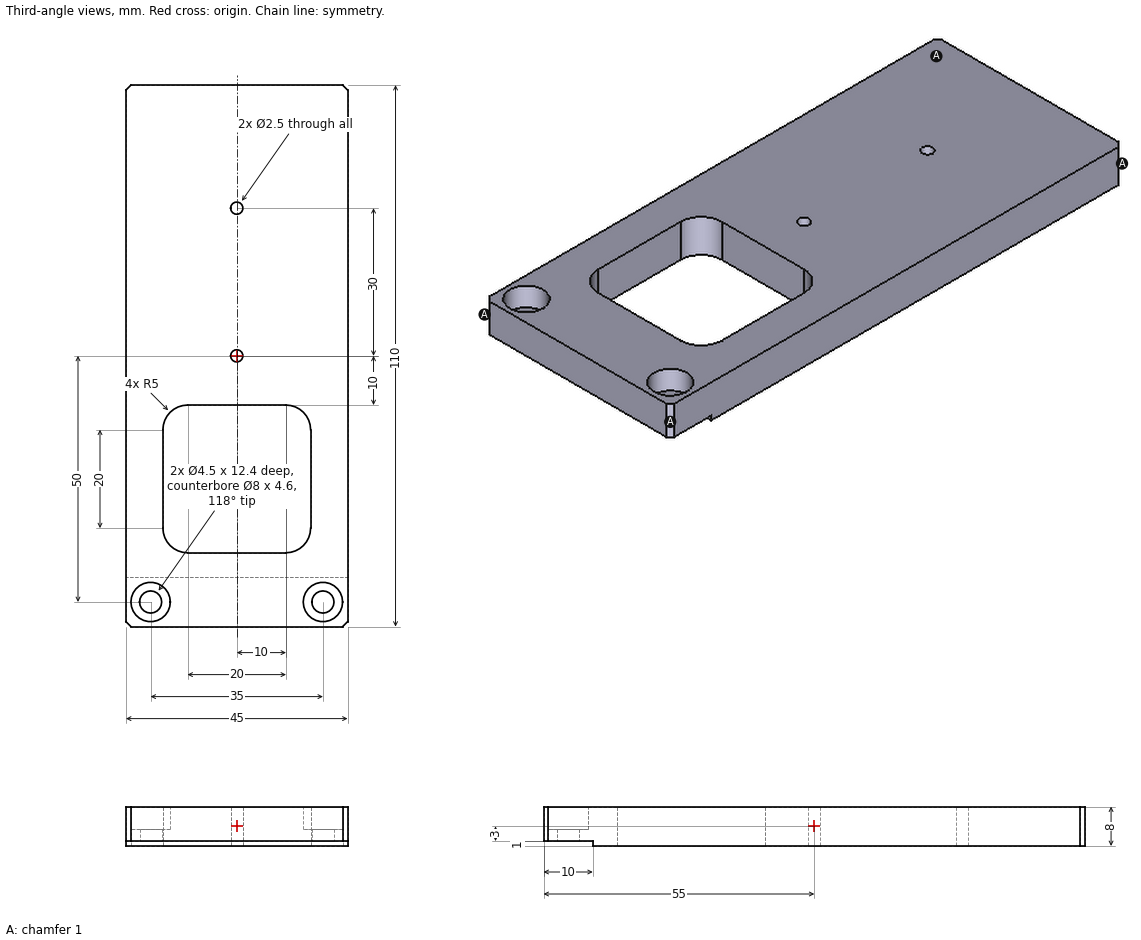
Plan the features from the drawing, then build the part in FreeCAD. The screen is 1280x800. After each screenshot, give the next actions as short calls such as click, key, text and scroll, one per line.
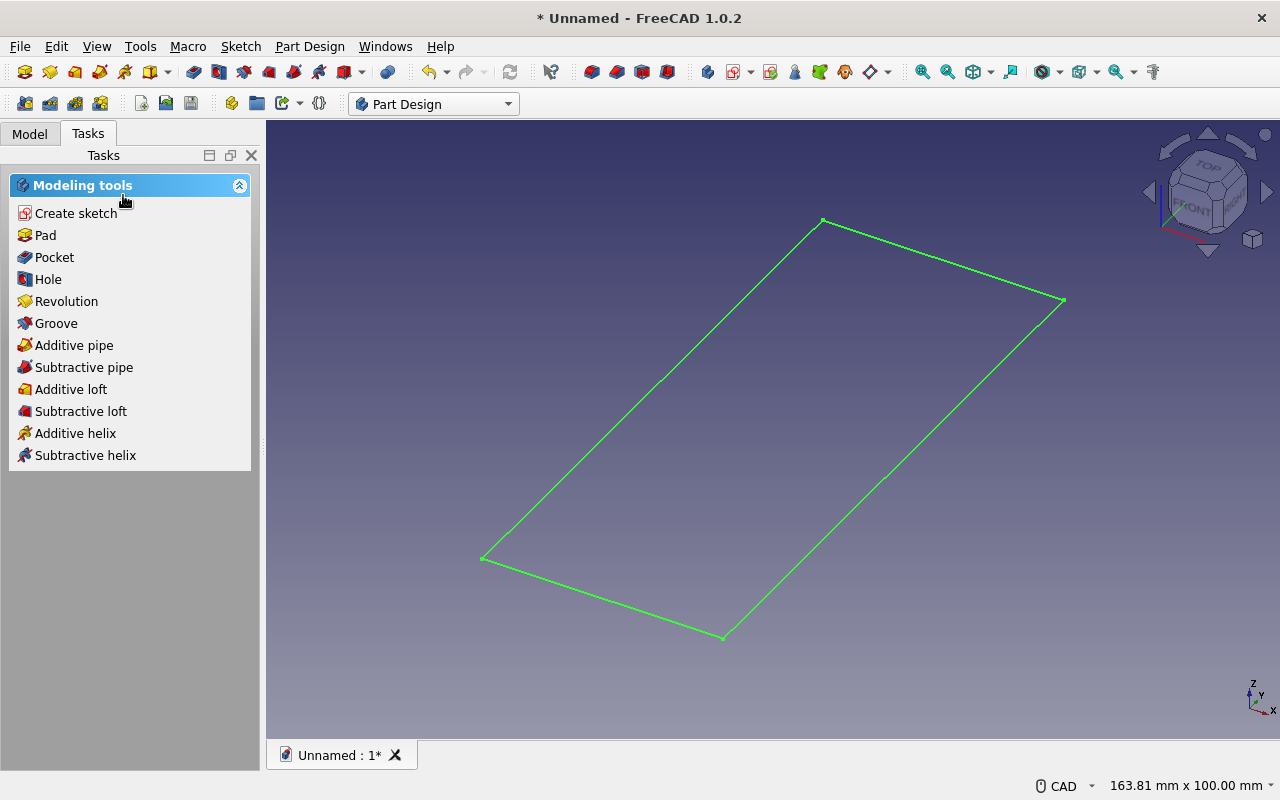
click(25, 72)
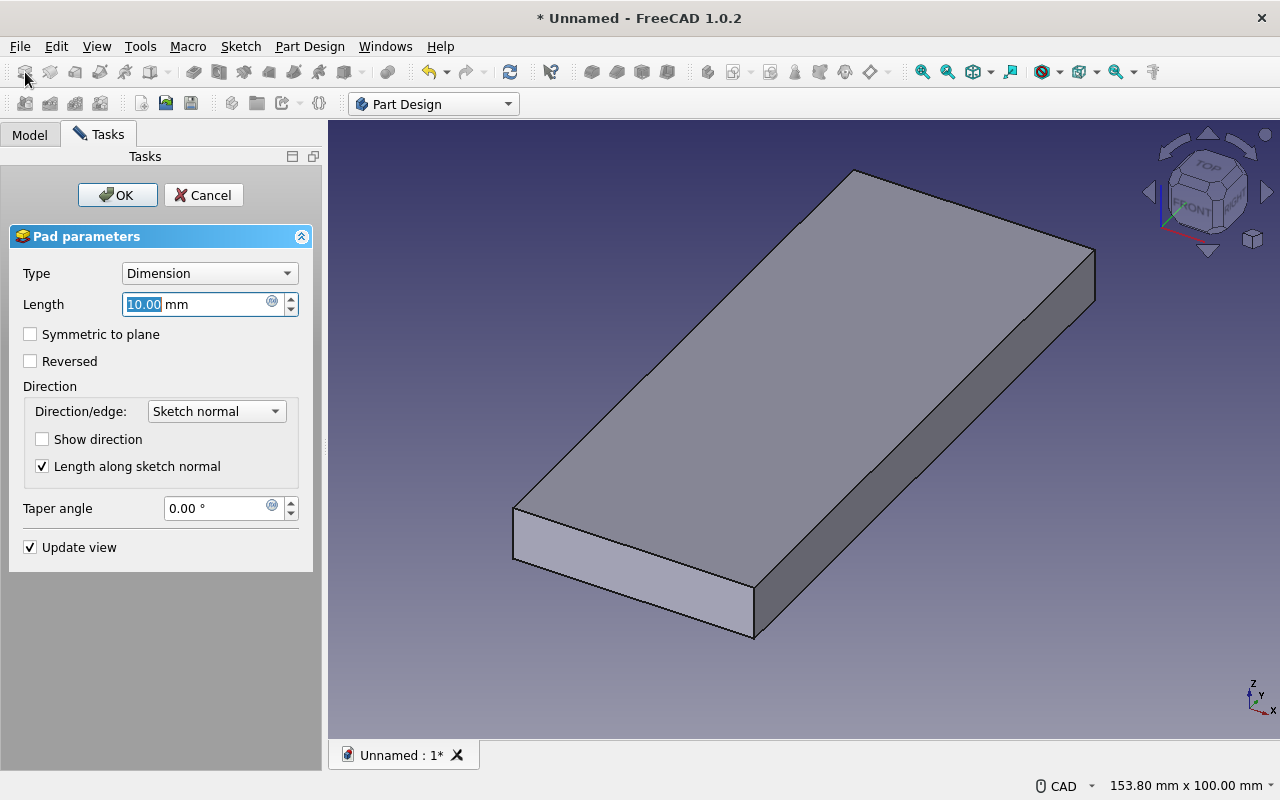
text(8)
key(Tab)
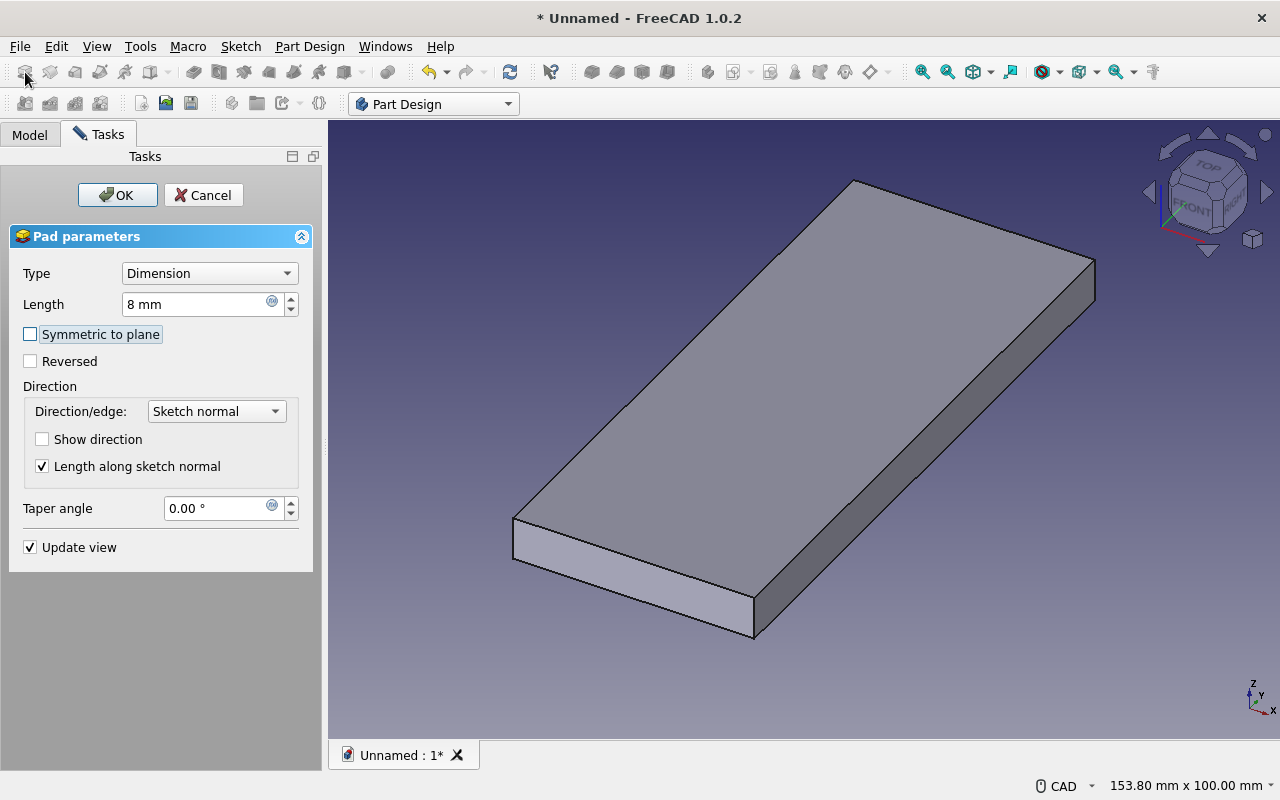
click(31, 334)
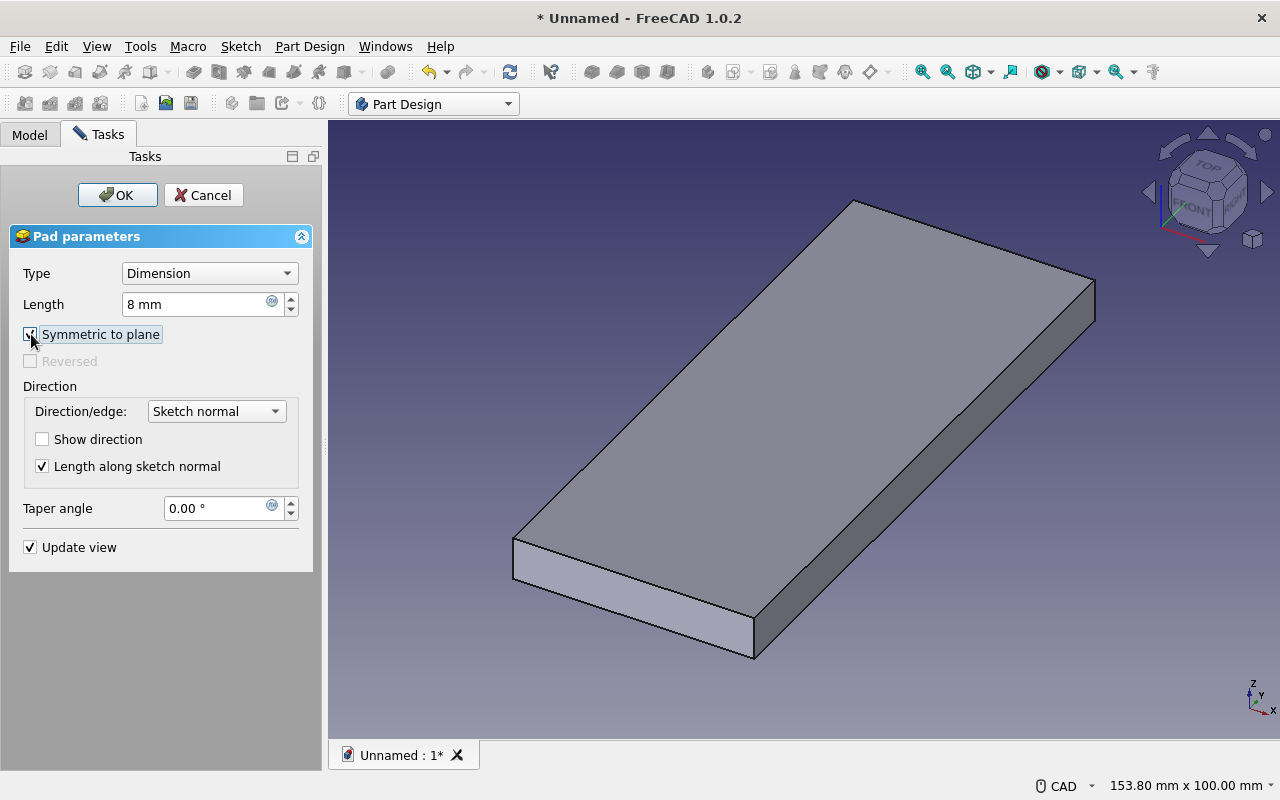
click(118, 195)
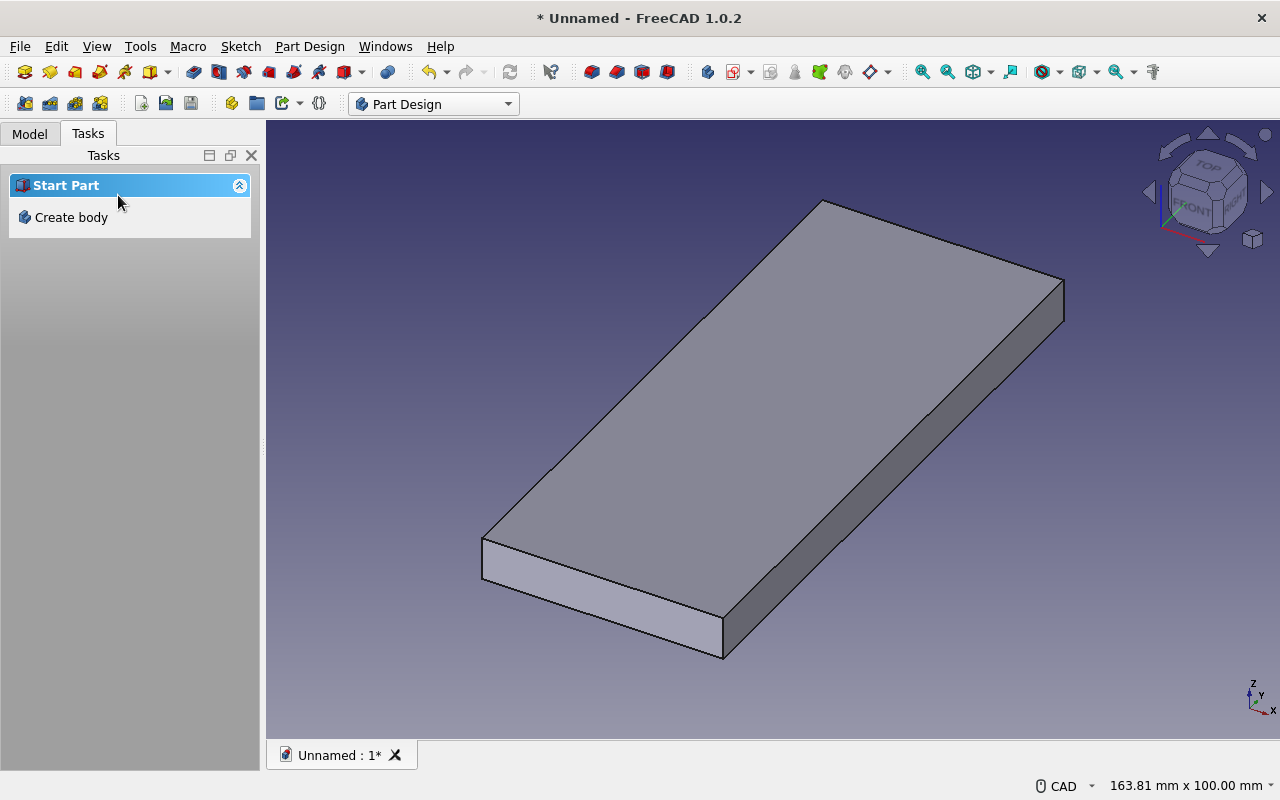
click(870, 312)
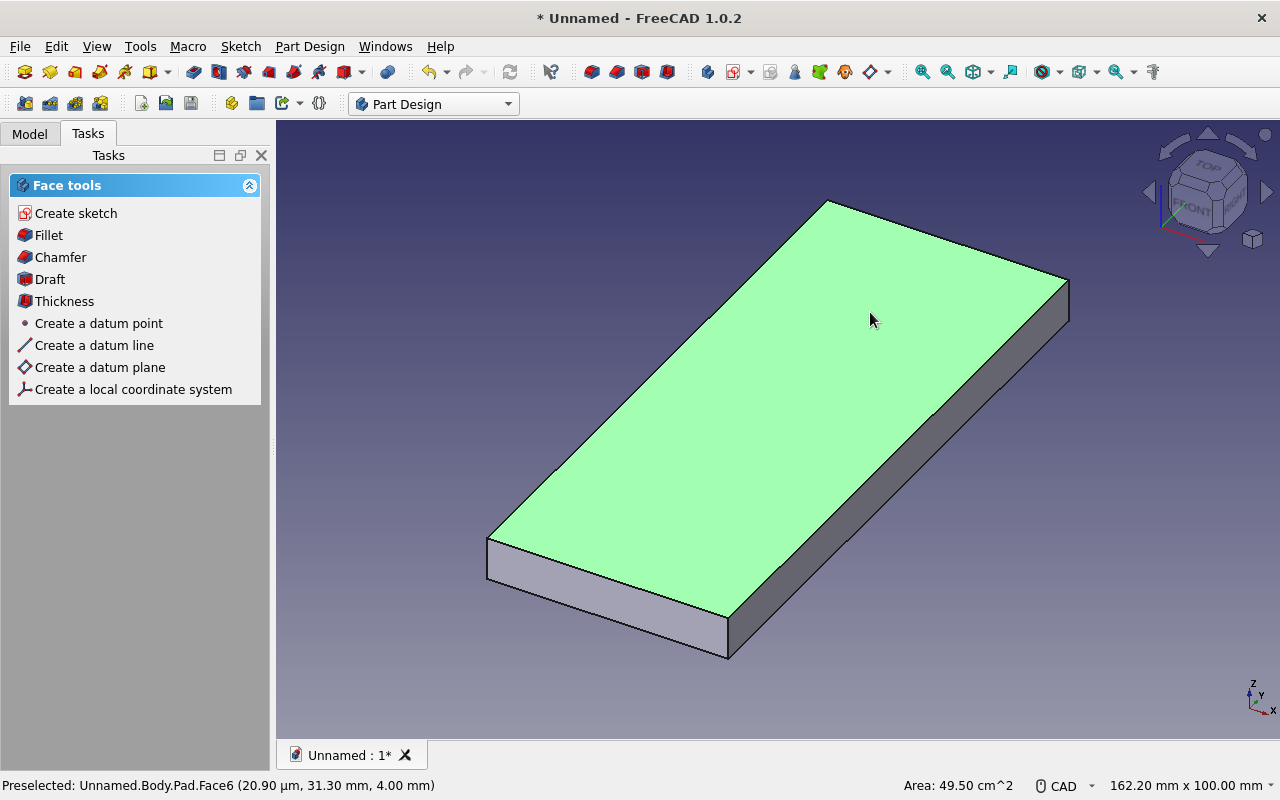
click(732, 72)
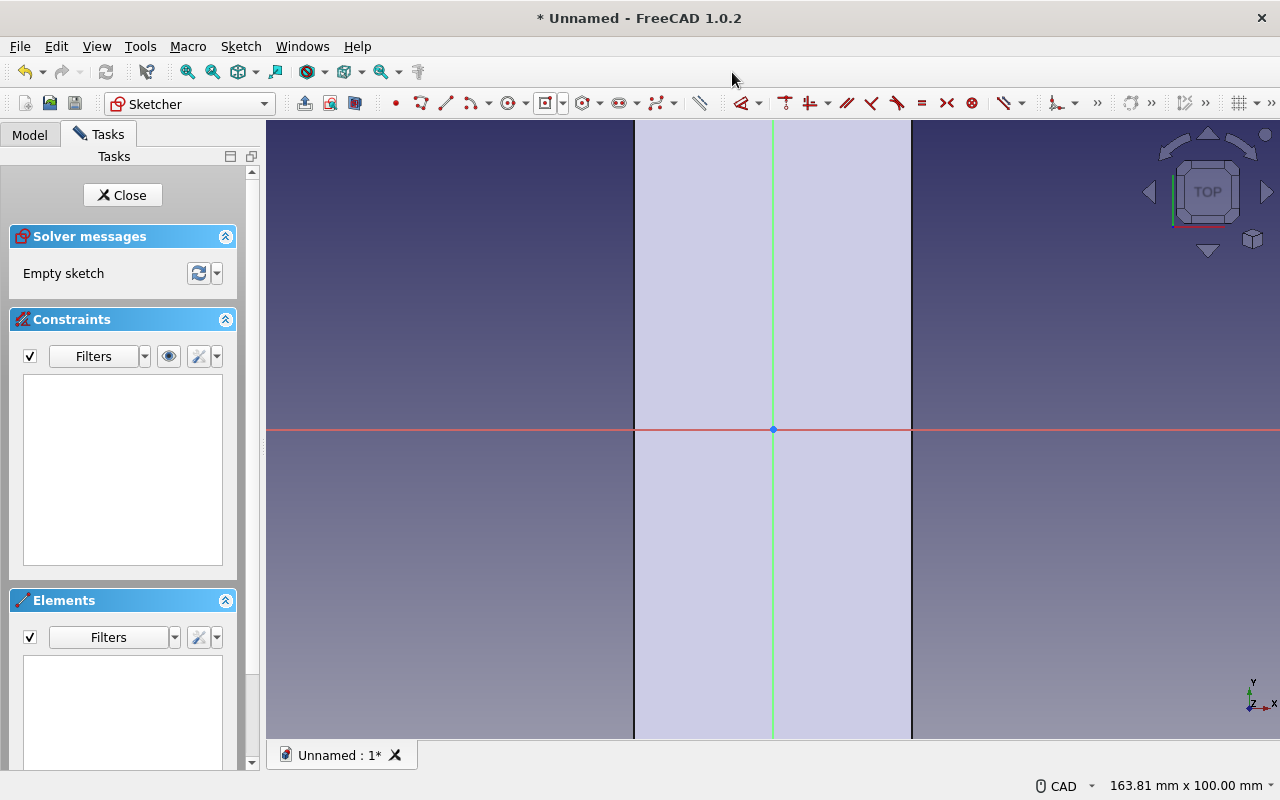
scroll(395, 148, down, 1)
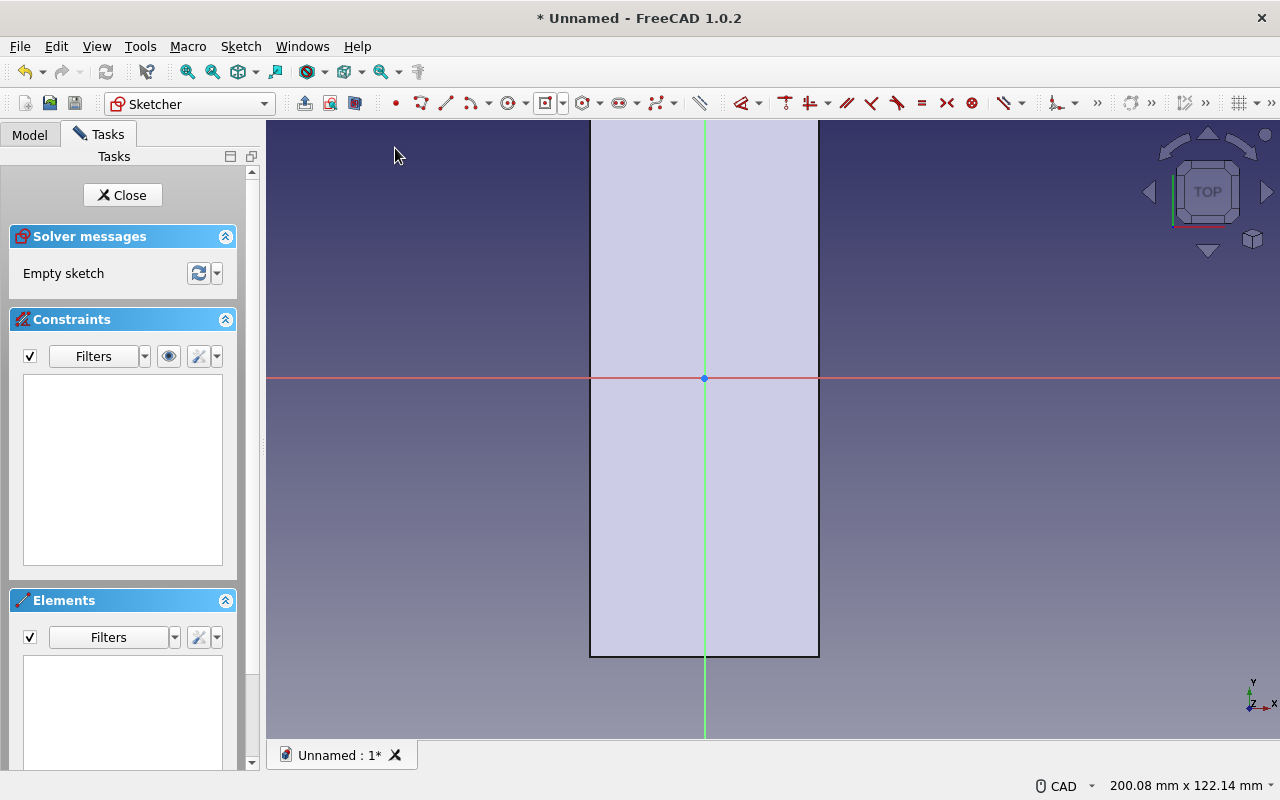
scroll(705, 676, up, 2)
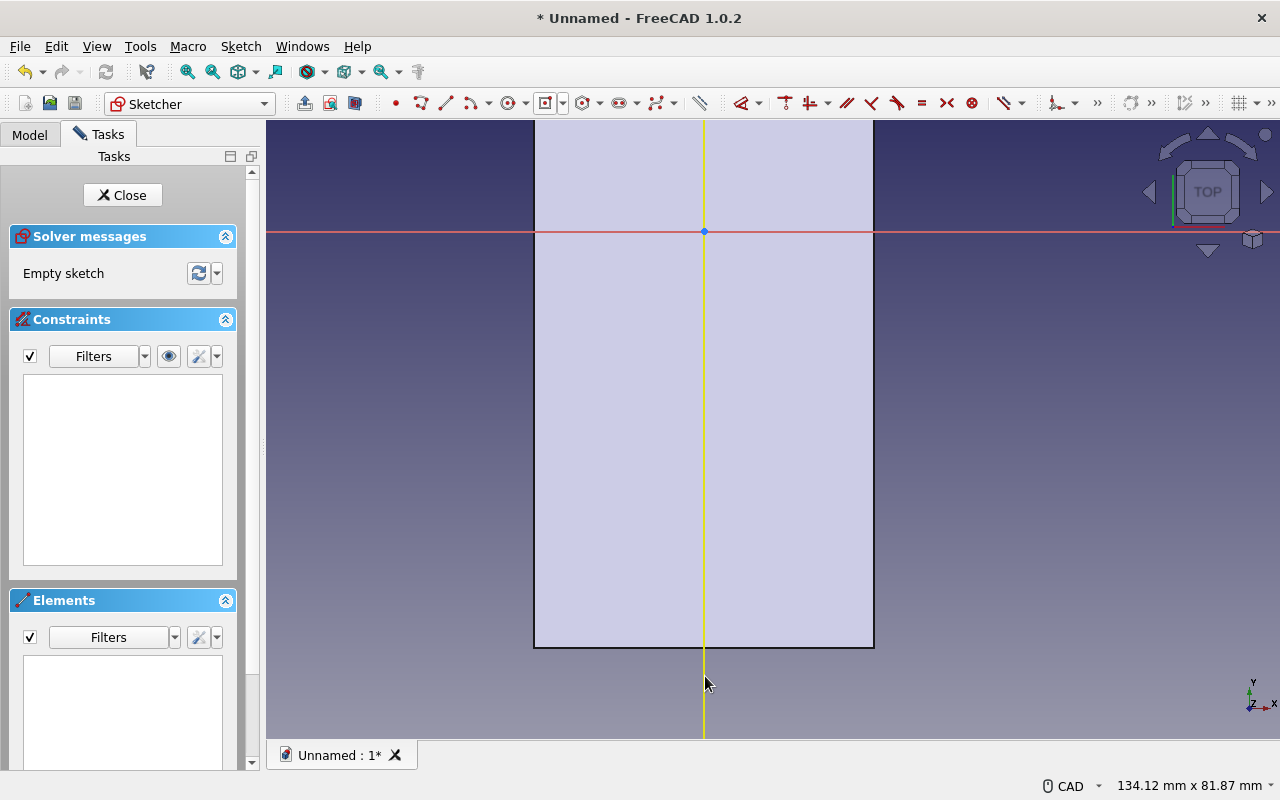
click(508, 104)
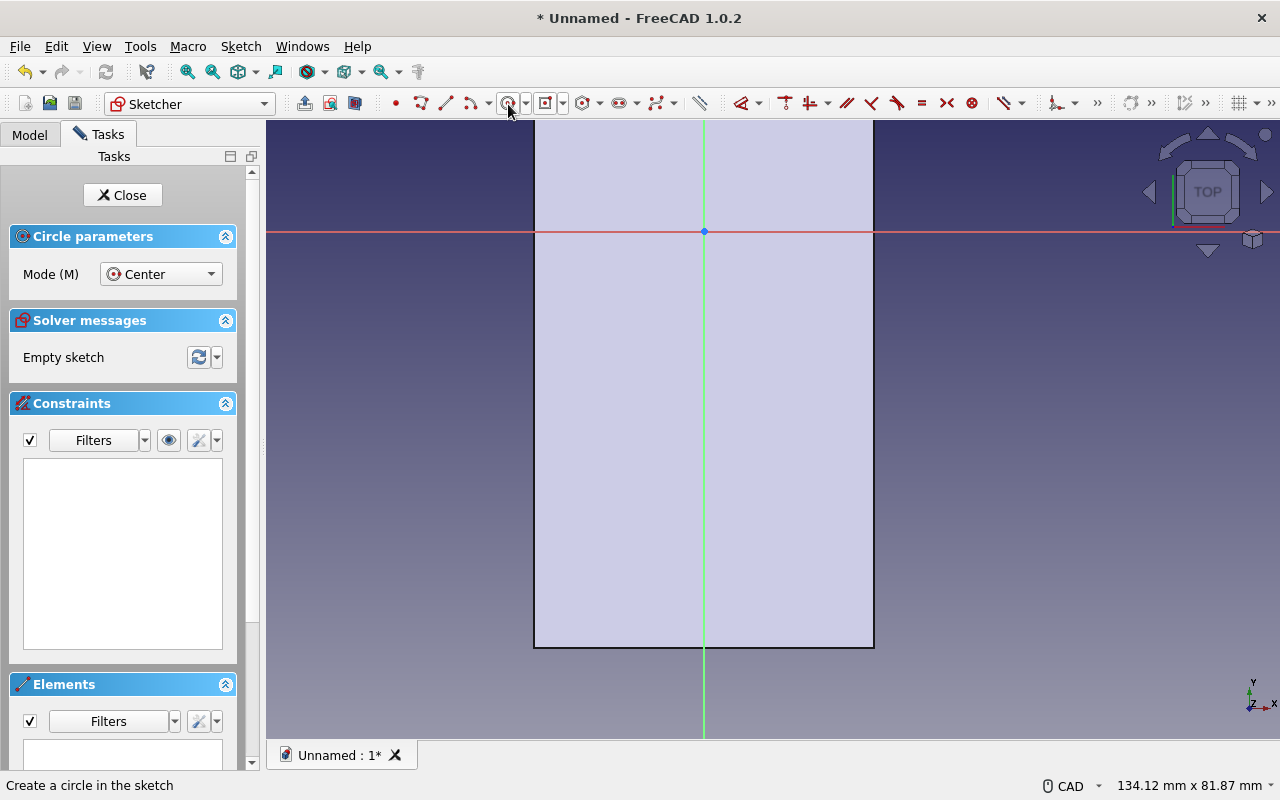
scroll(572, 610, up, 2)